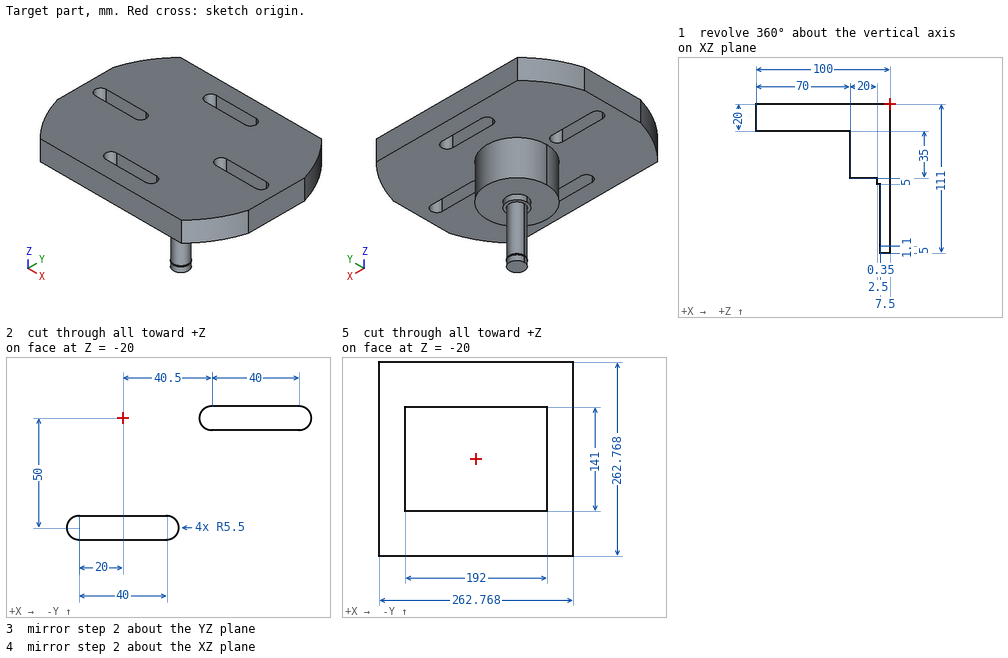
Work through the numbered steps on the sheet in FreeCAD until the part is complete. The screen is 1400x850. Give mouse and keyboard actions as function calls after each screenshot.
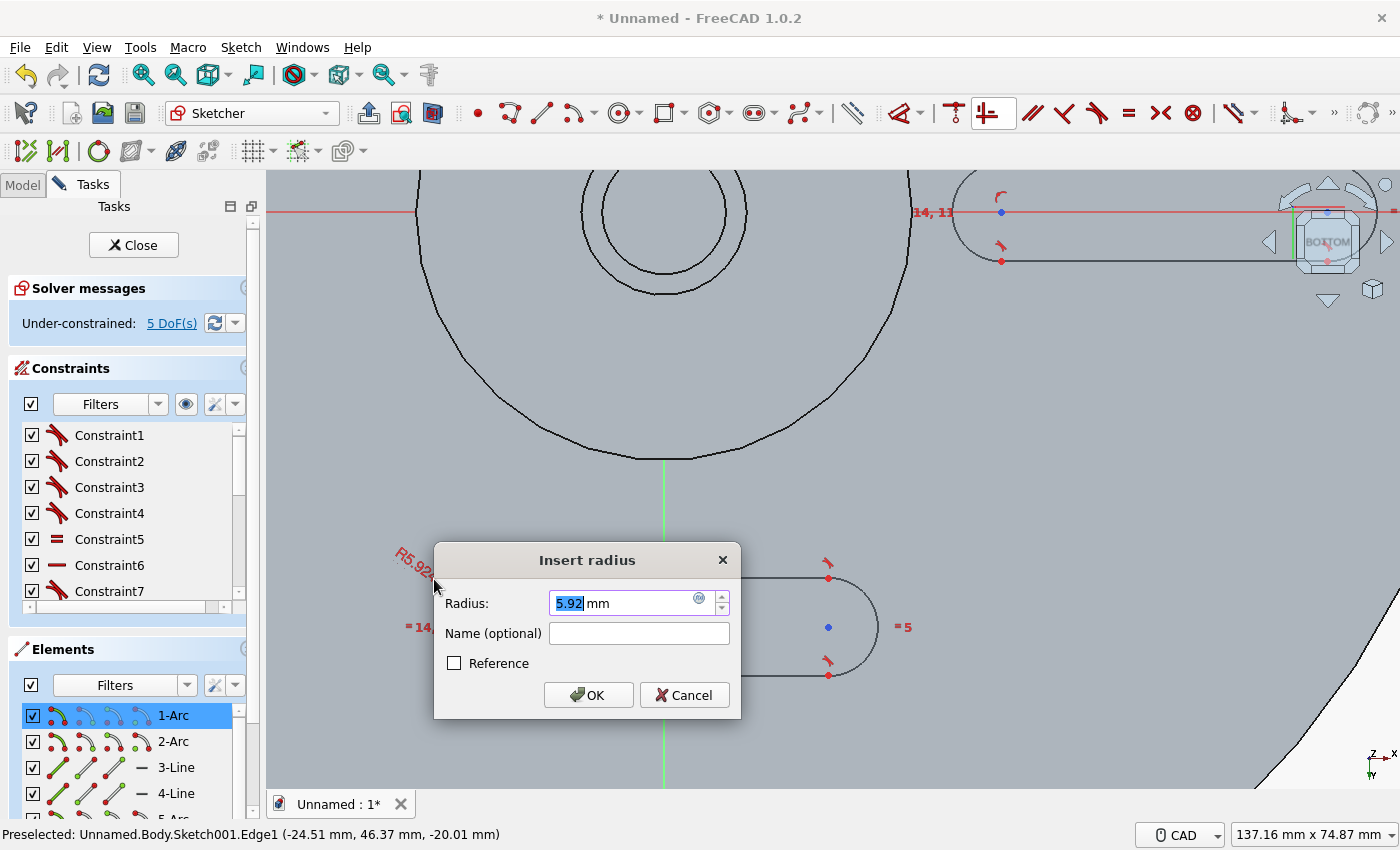
text(5.5)
key(Return)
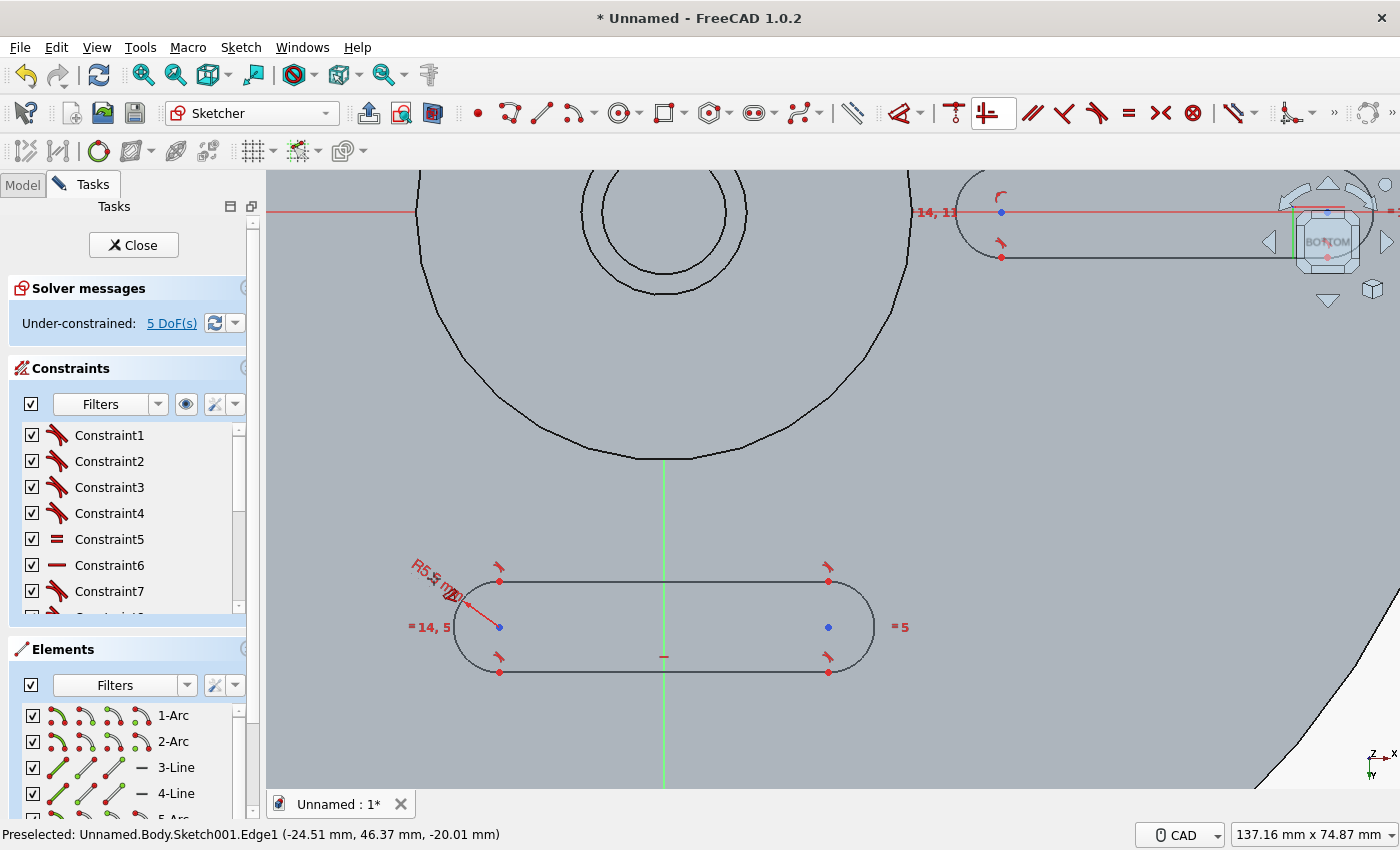
click(598, 582)
click(588, 616)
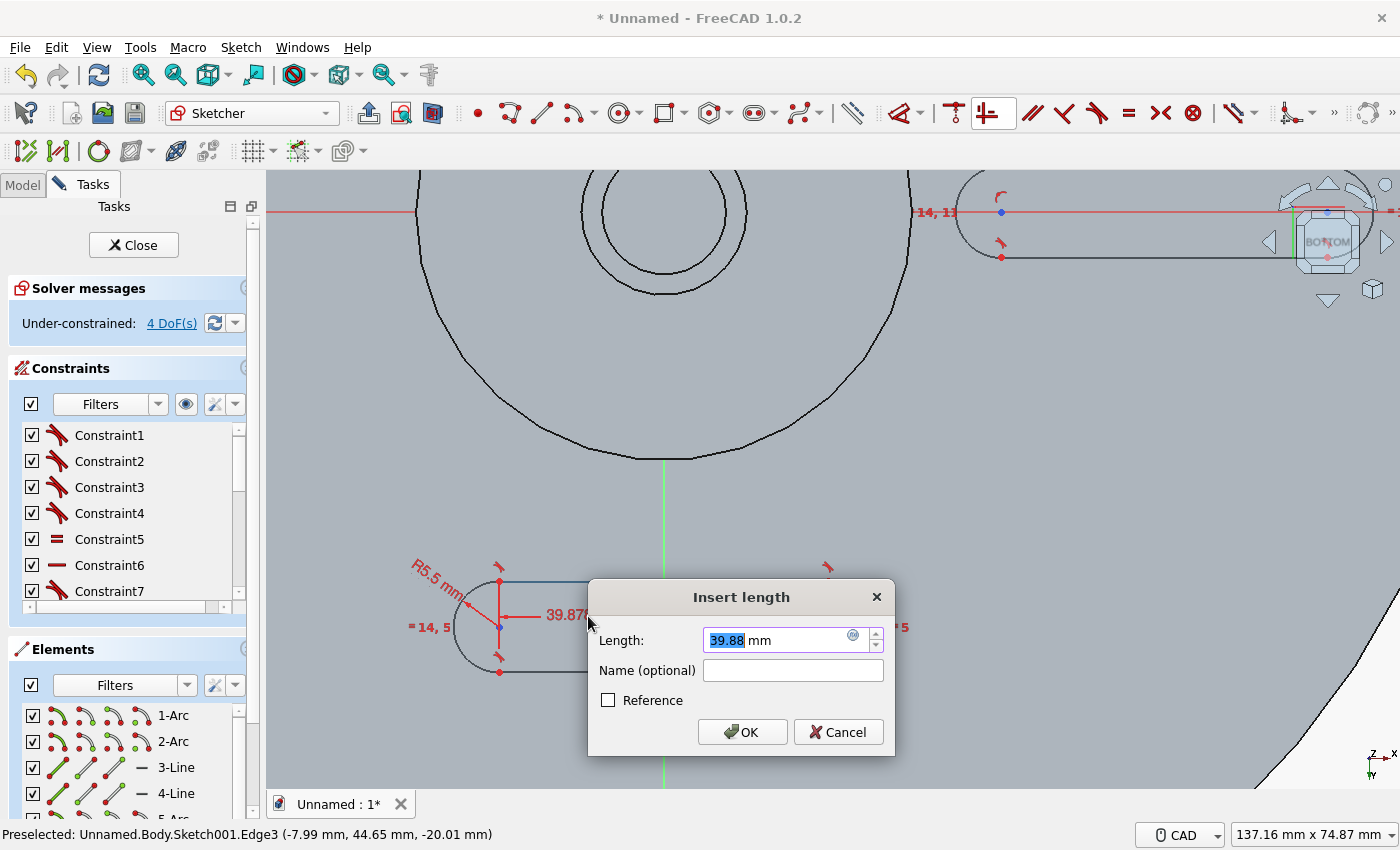
text(40)
key(Return)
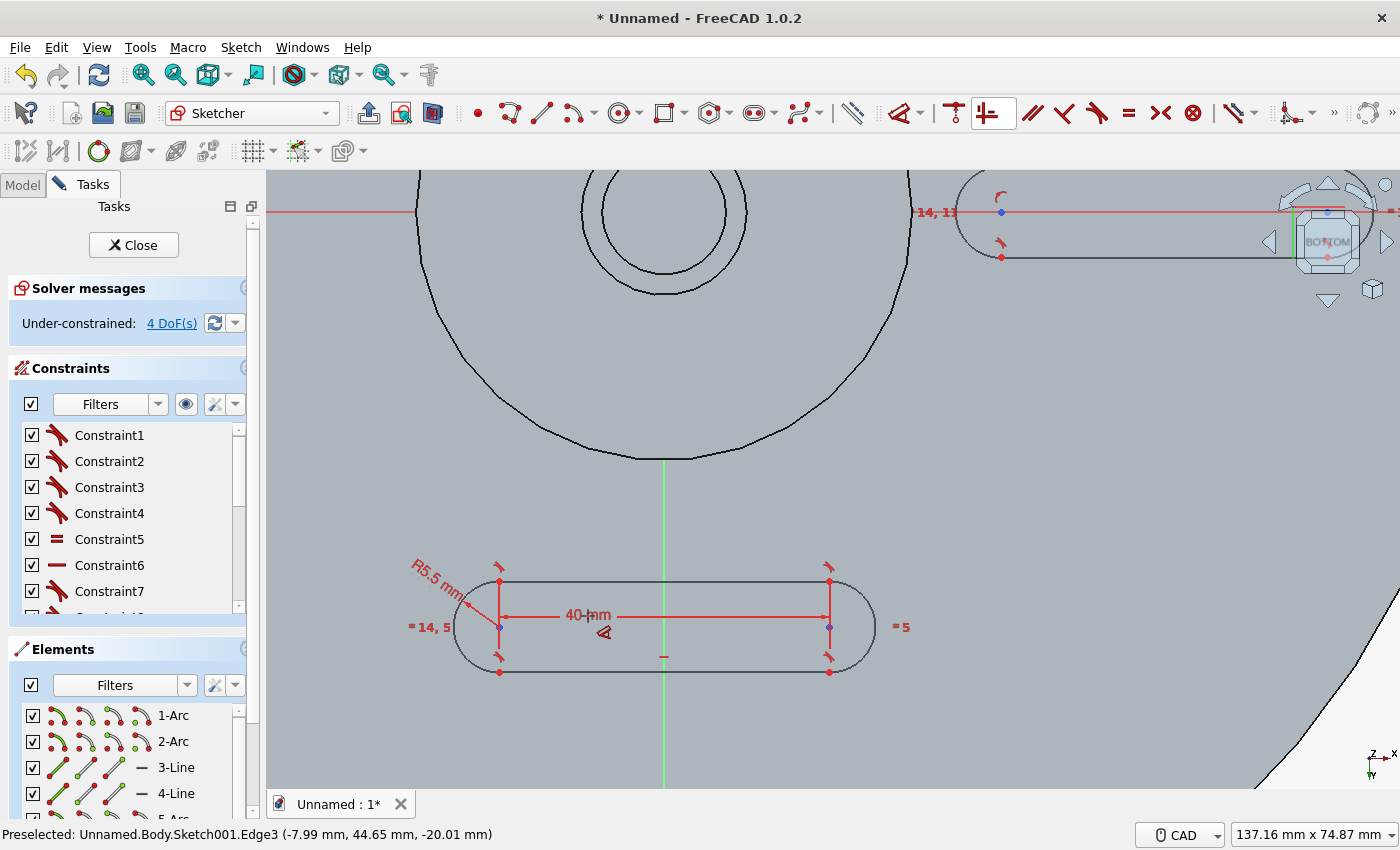
scroll(460, 602, down, 2)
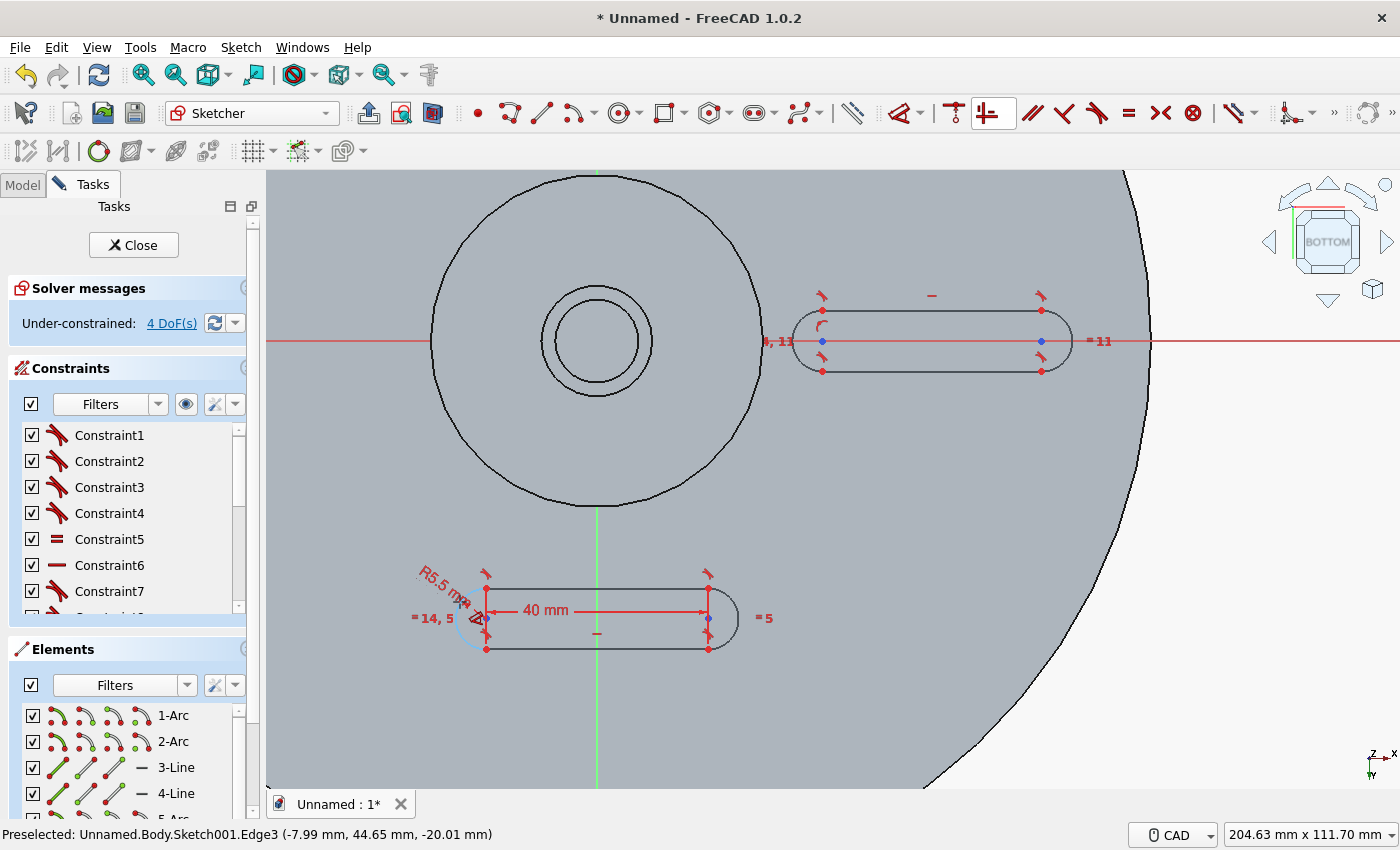
click(889, 311)
click(932, 277)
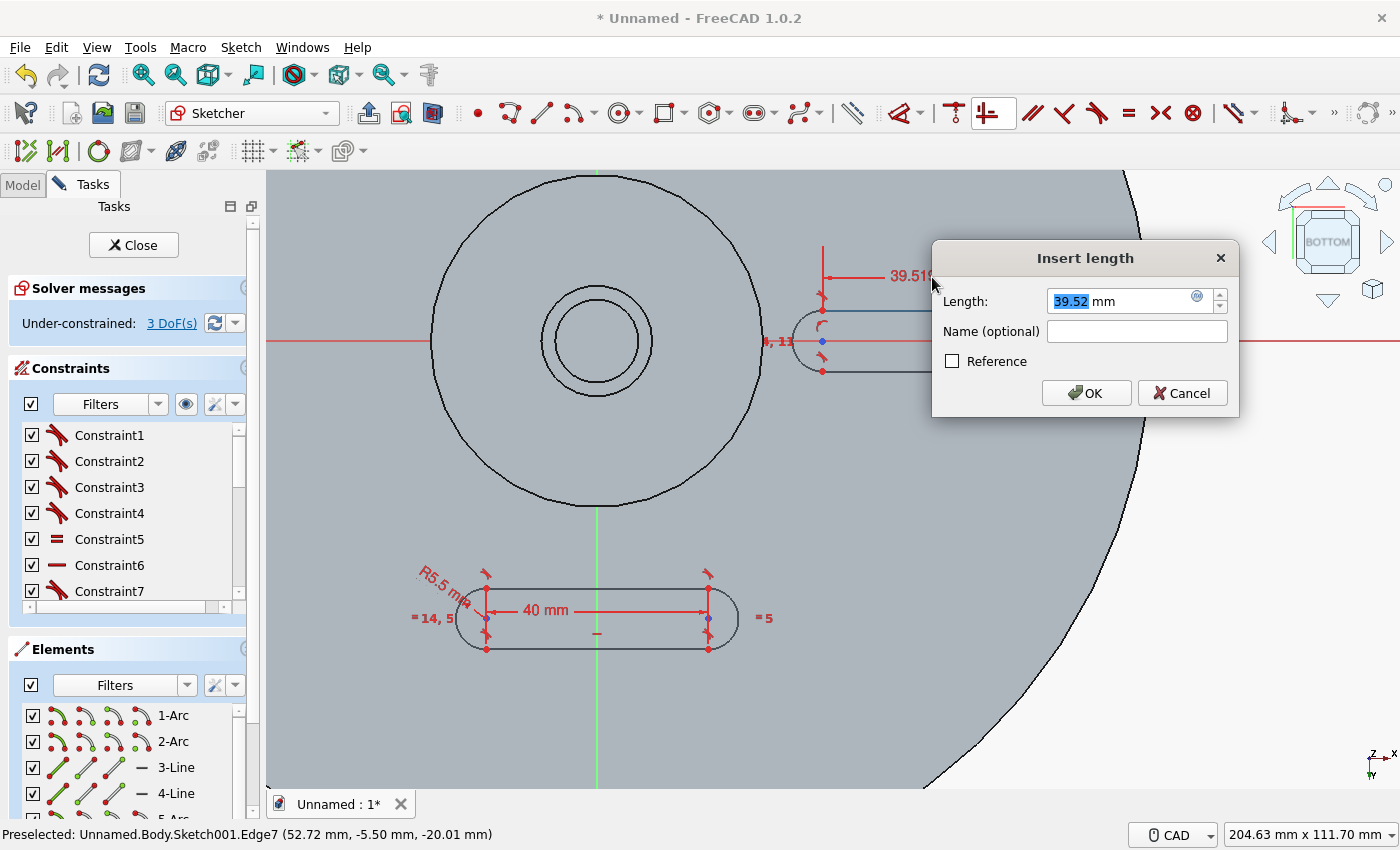
text(40)
key(Return)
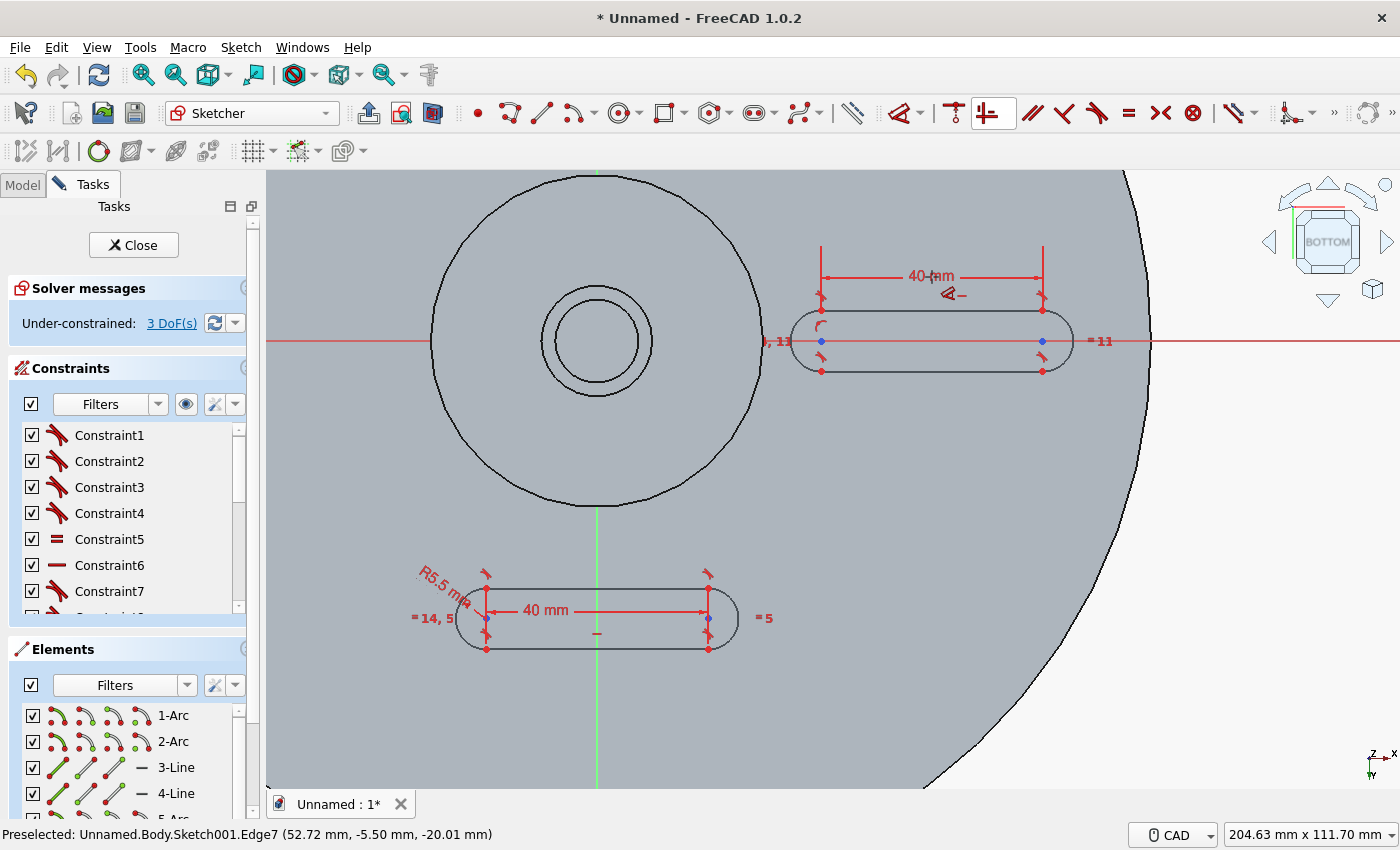
click(486, 589)
click(542, 307)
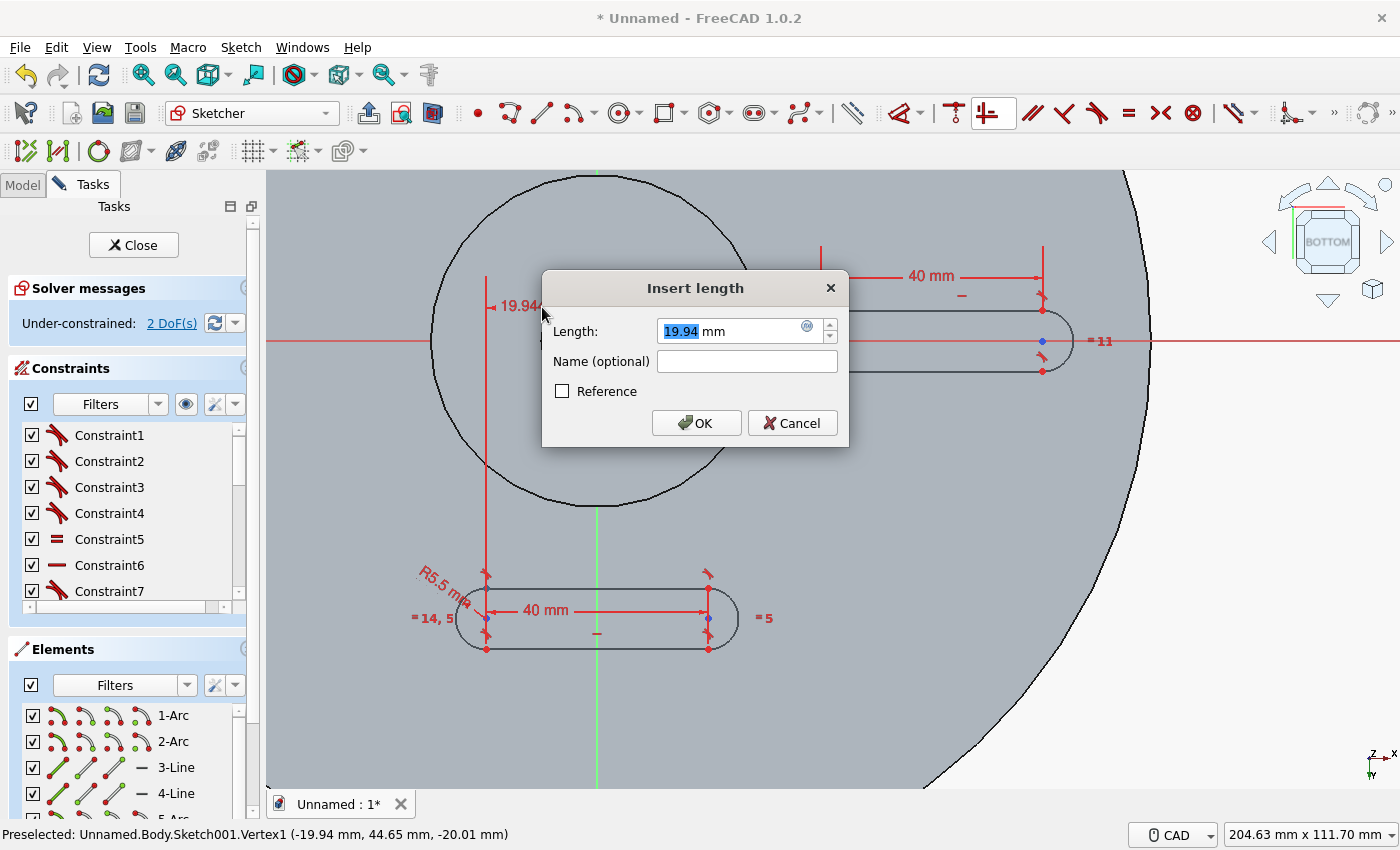
text(20)
key(Return)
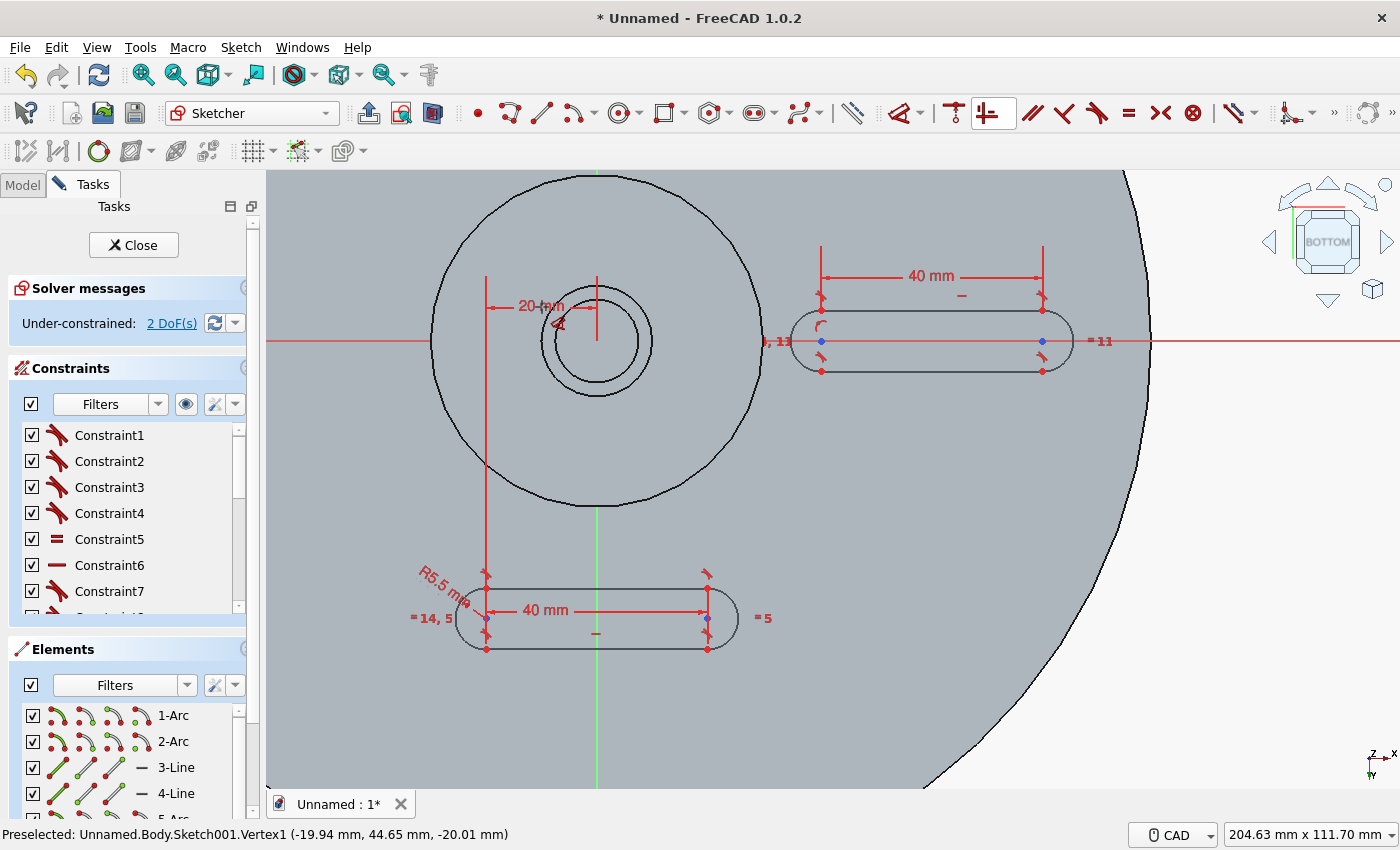
click(486, 619)
click(452, 480)